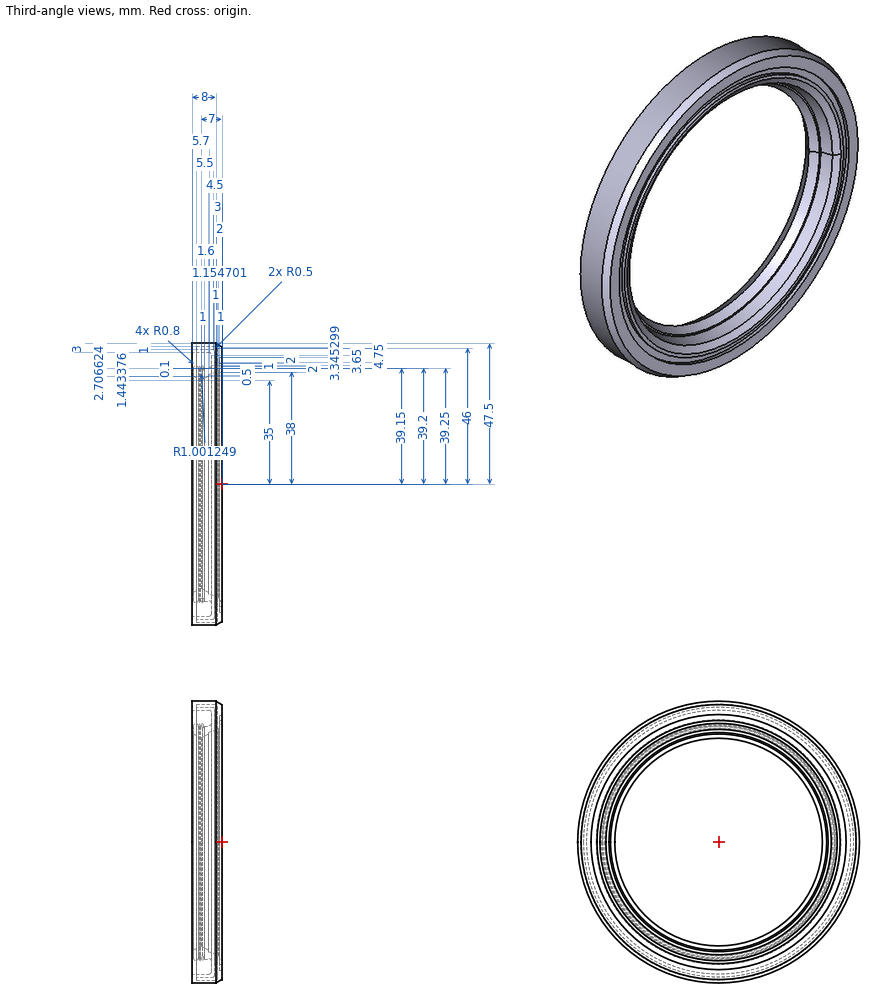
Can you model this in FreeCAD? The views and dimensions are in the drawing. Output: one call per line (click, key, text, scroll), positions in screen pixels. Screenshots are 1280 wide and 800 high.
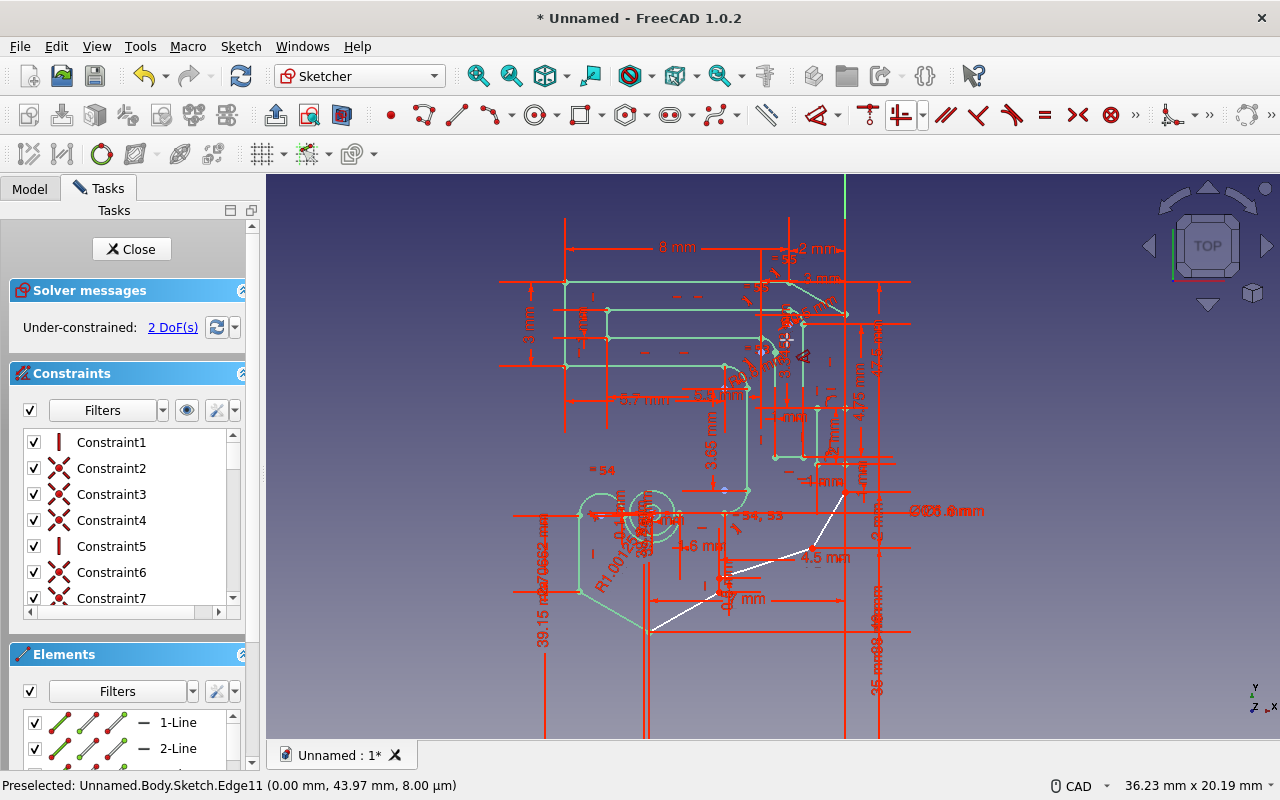
scroll(813, 548, up, 2)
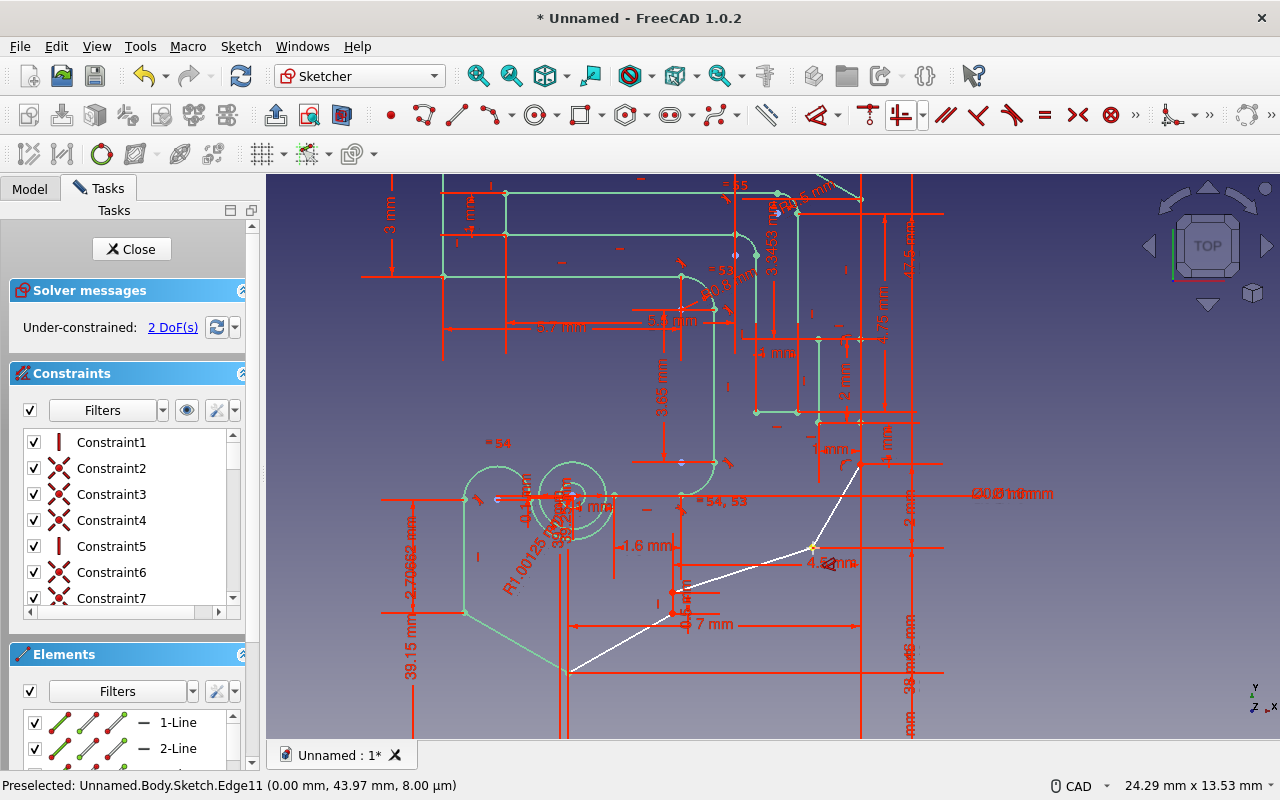
click(812, 548)
click(825, 490)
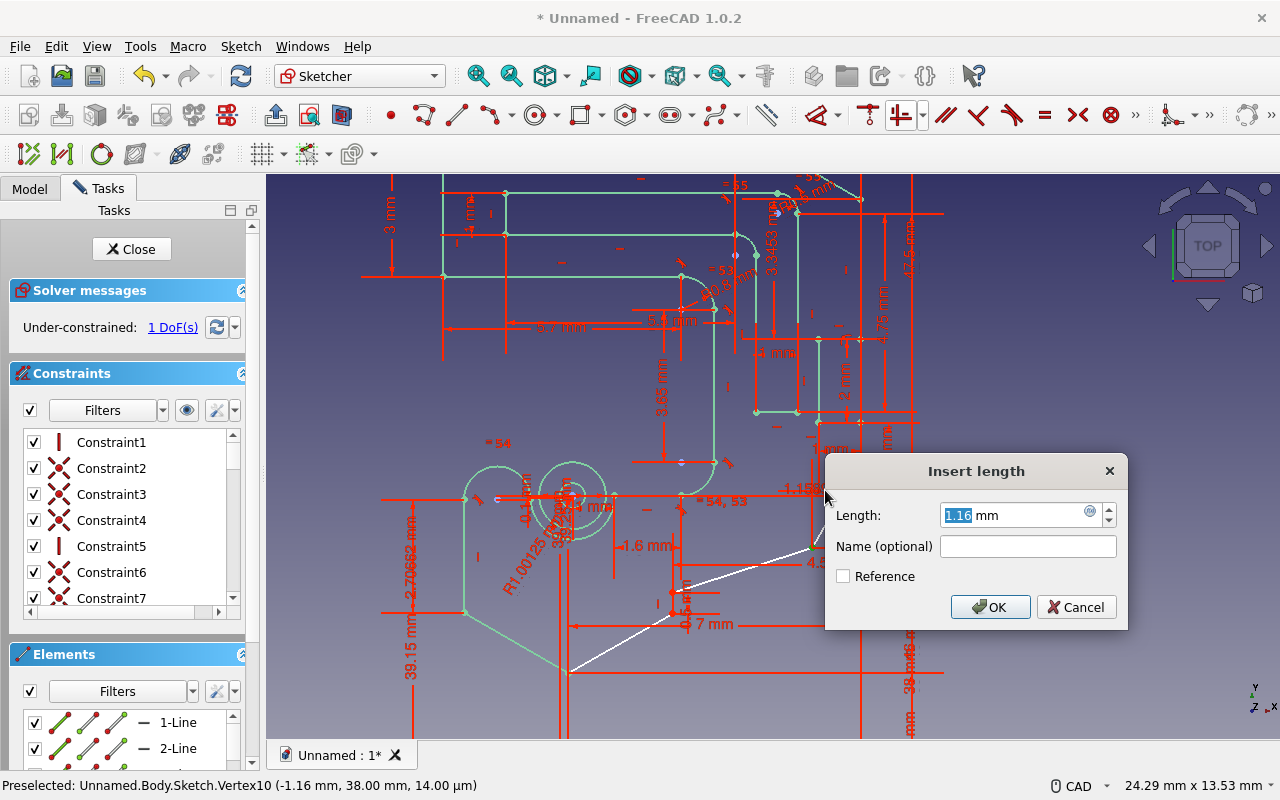
text(1.154701)
key(Return)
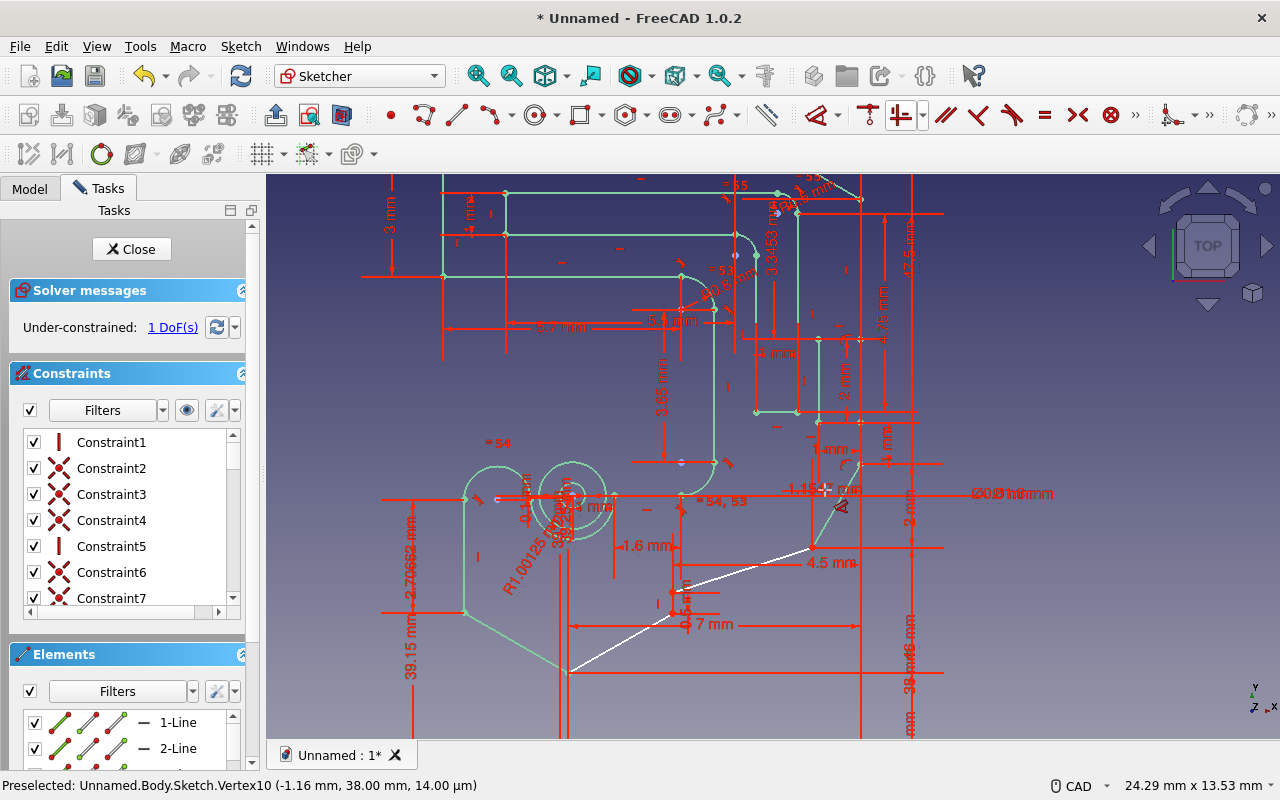
click(600, 655)
click(534, 630)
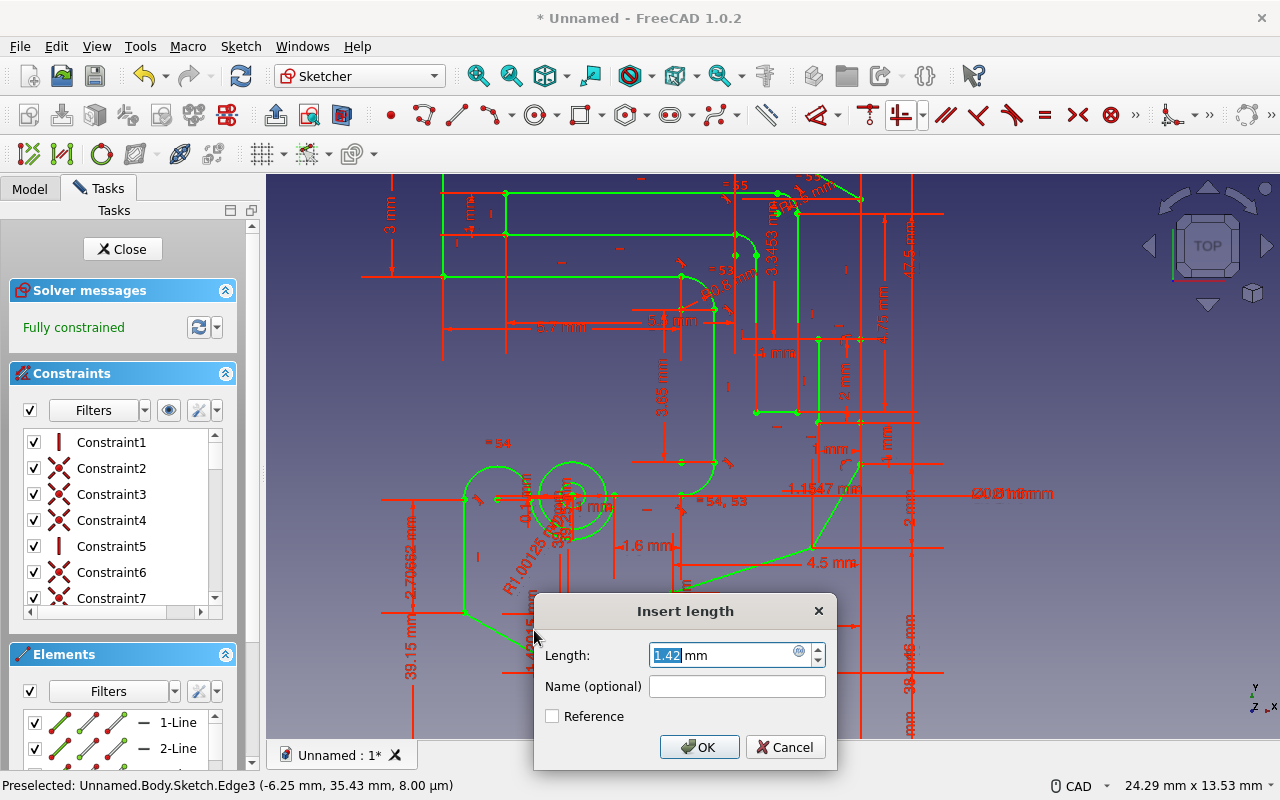
text(1.443376)
key(Return)
key(Escape)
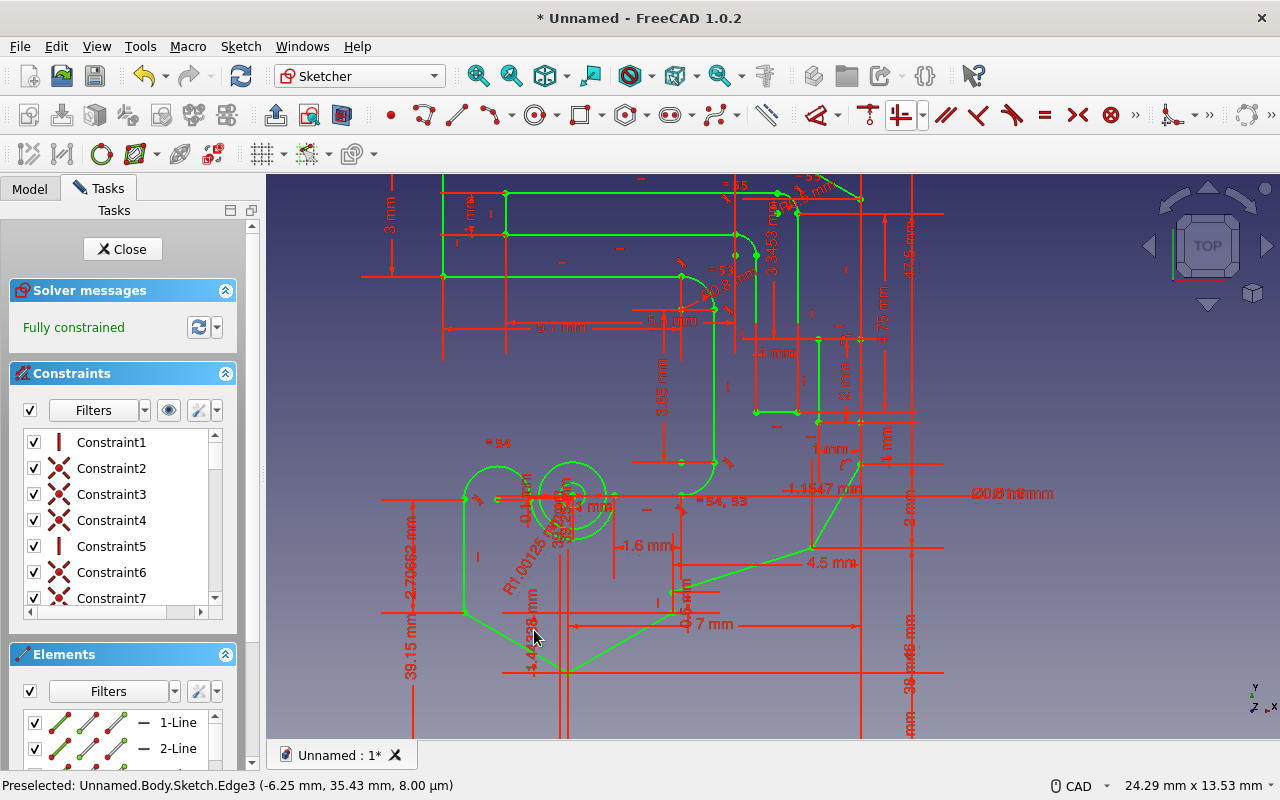
click(123, 249)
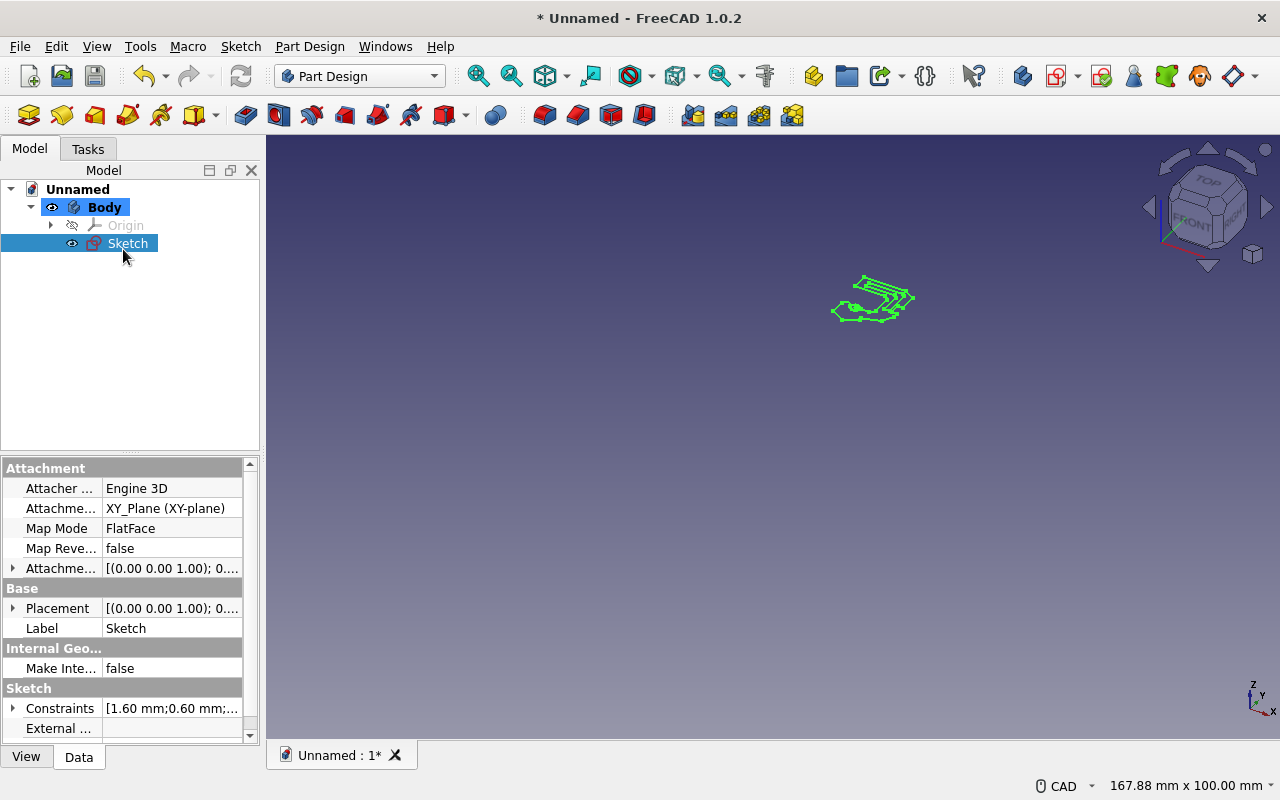
click(62, 116)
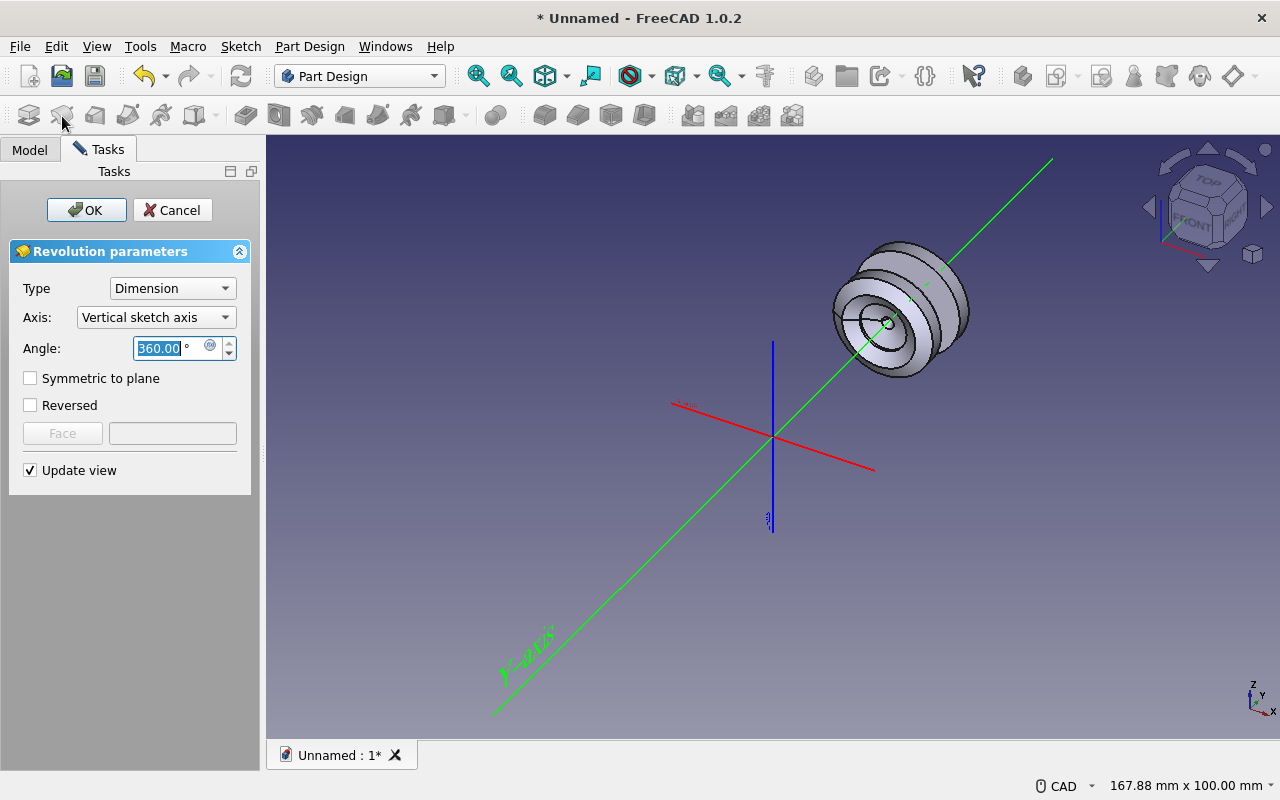
click(157, 318)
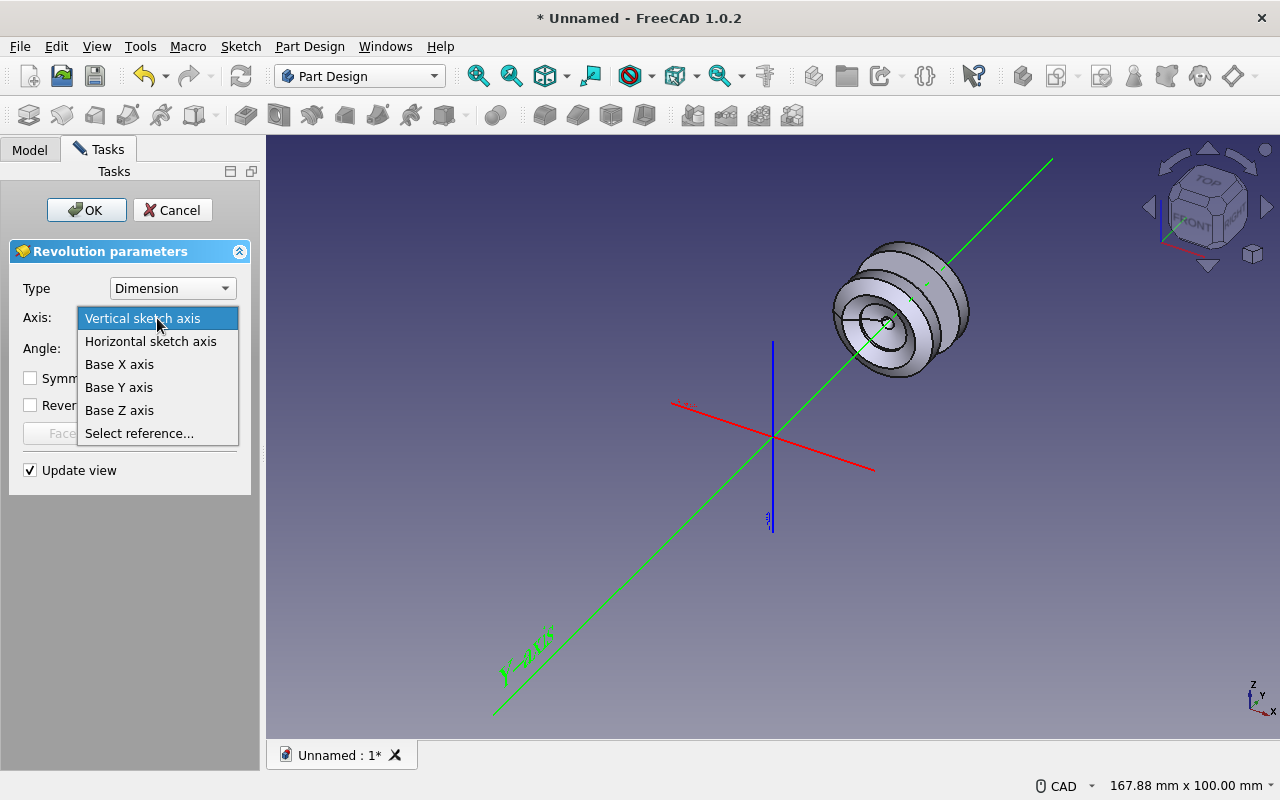
click(156, 342)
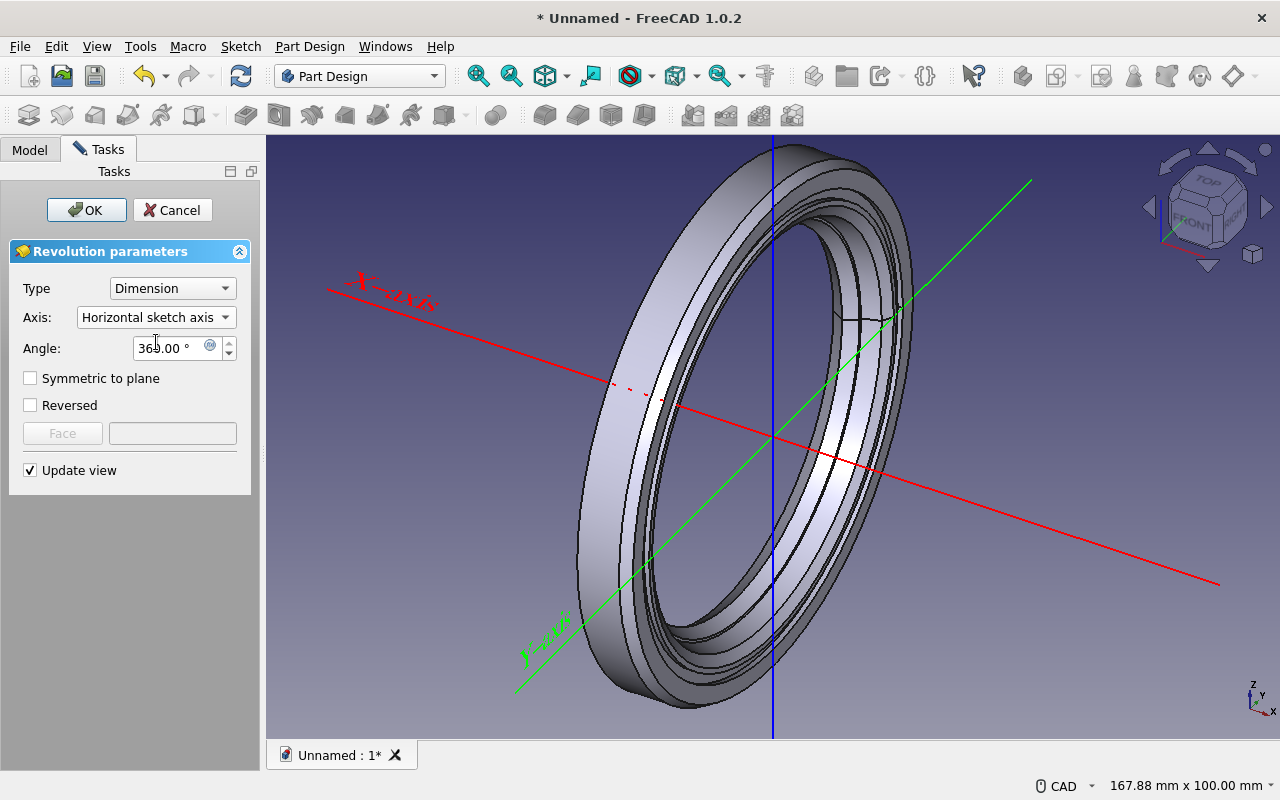
click(87, 210)